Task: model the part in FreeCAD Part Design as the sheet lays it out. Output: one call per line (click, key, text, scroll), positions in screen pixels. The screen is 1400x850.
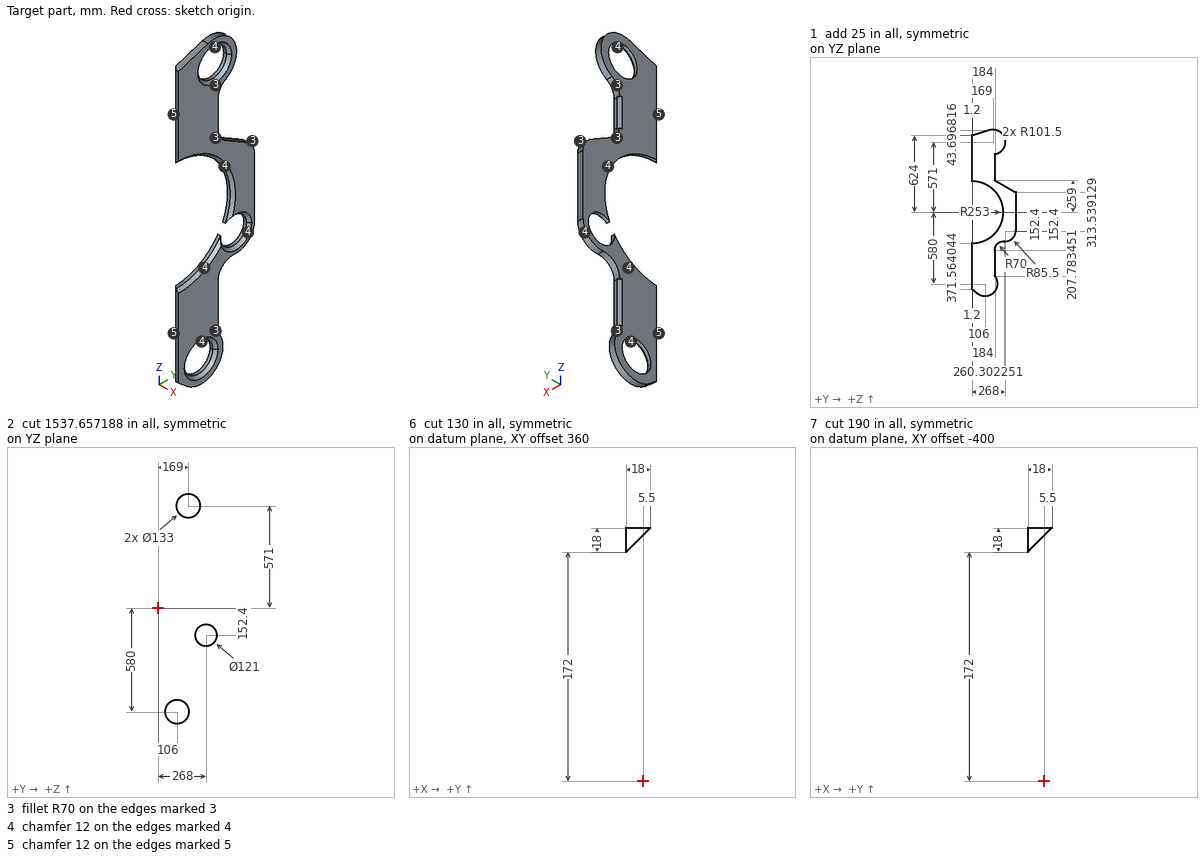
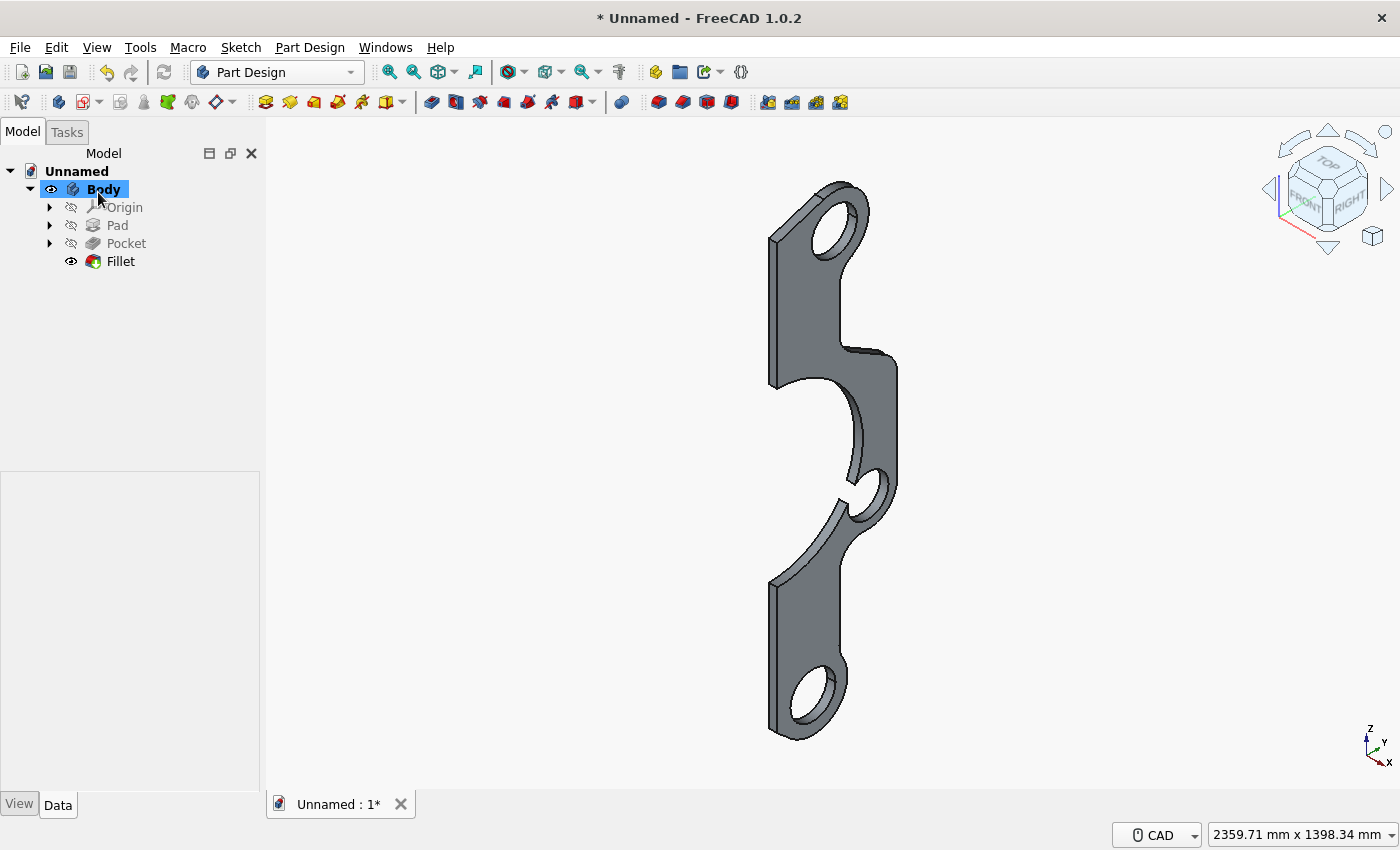
click(849, 392)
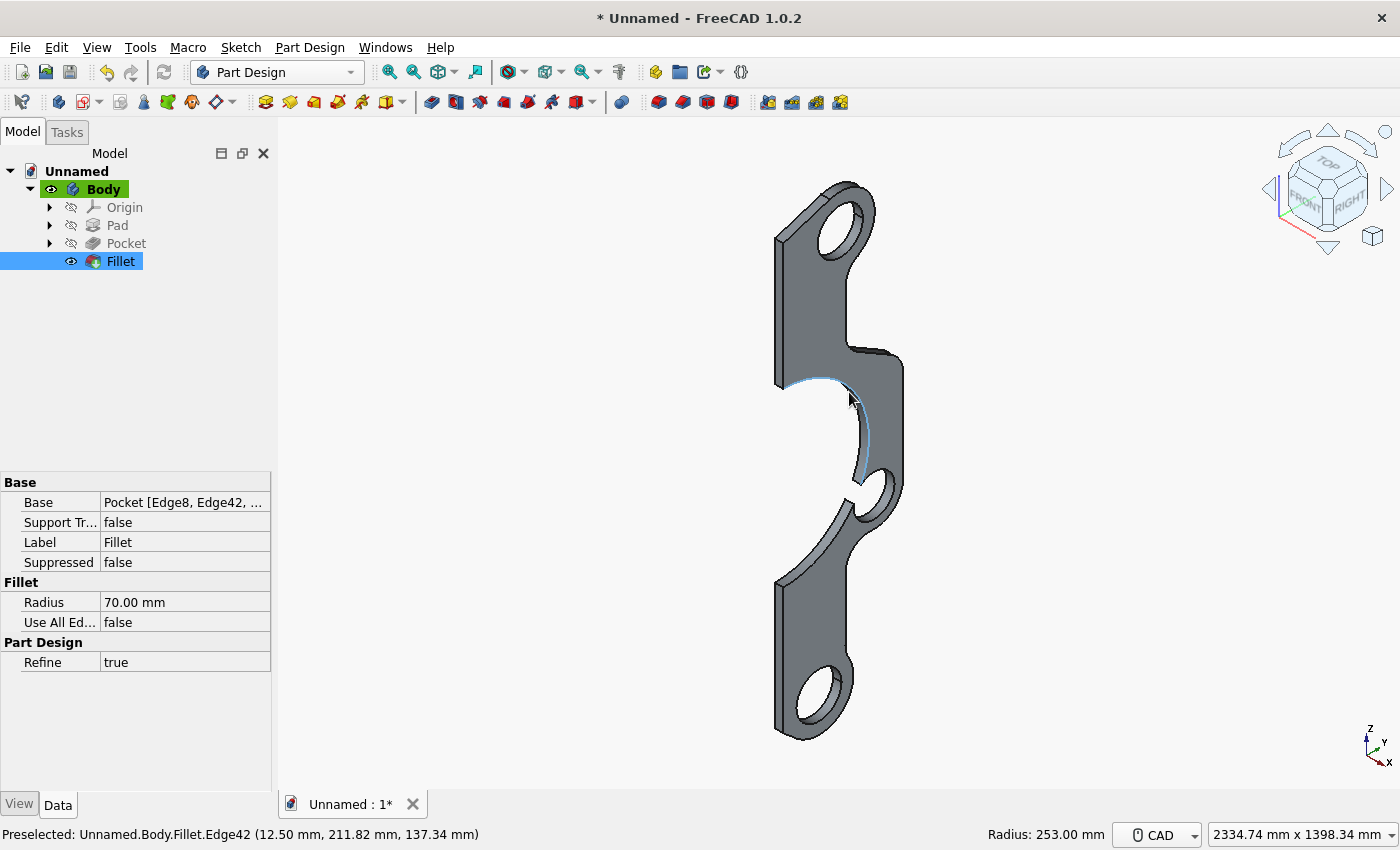
click(823, 552, ctrl)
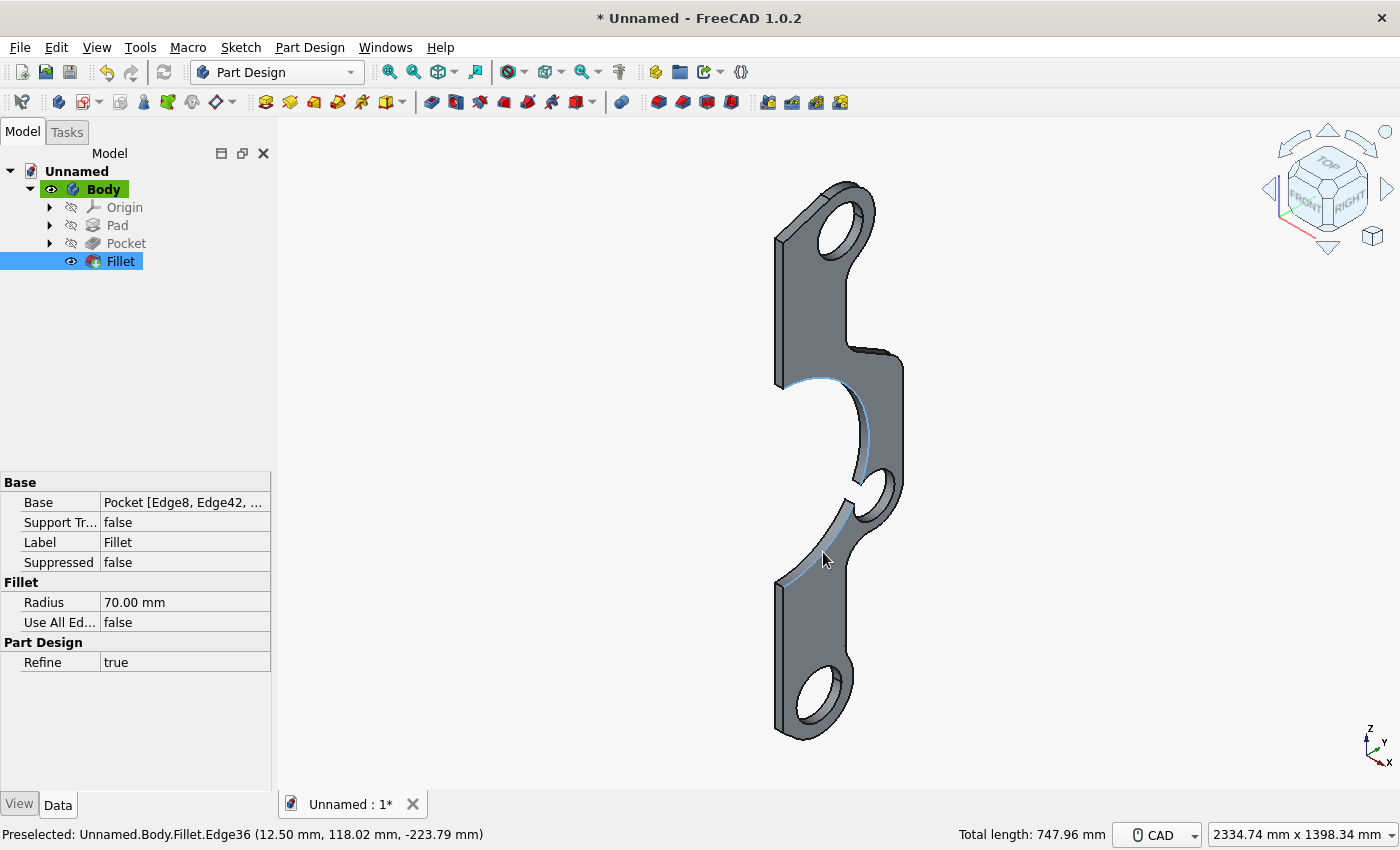
click(873, 519, ctrl)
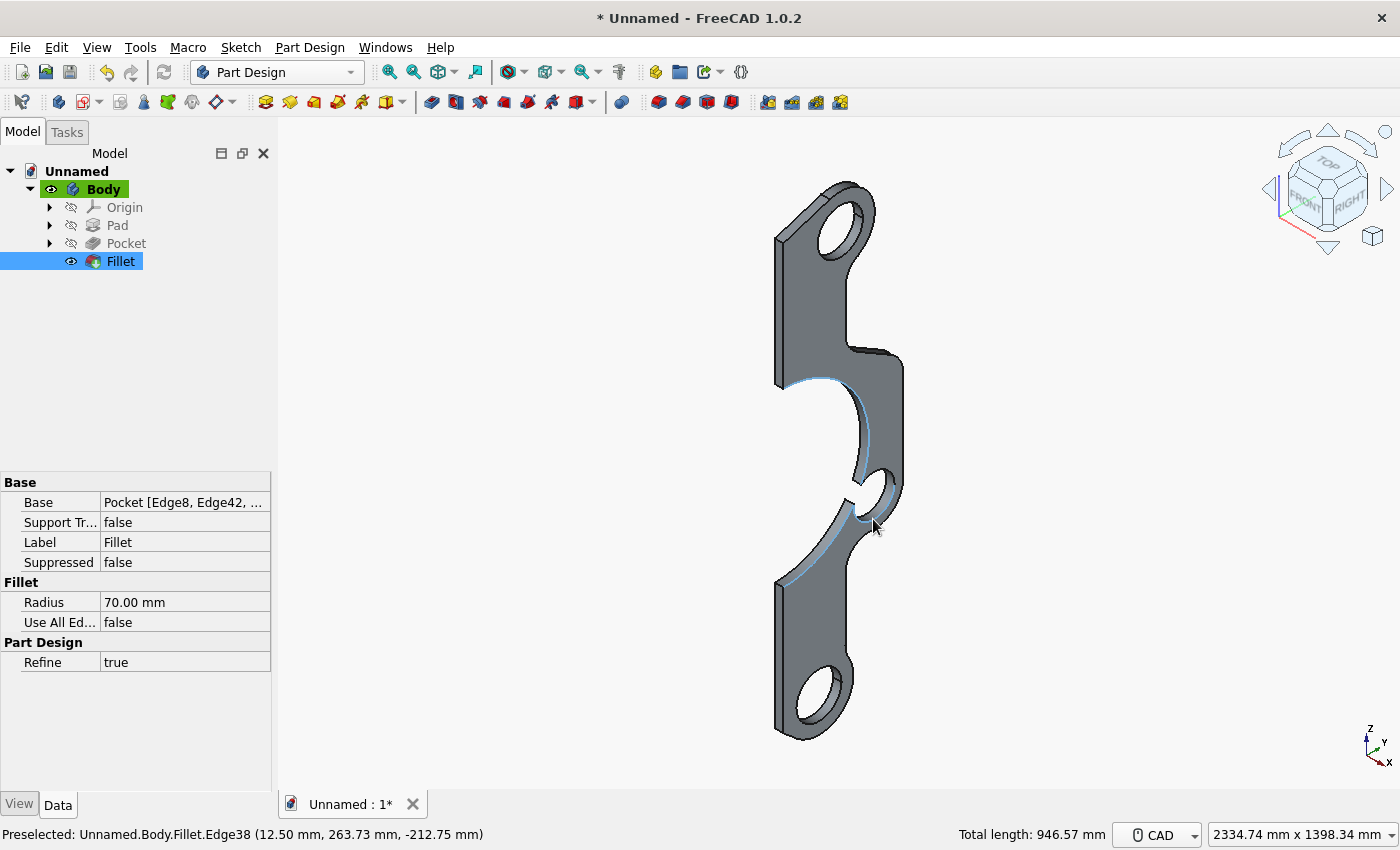
click(833, 259, ctrl)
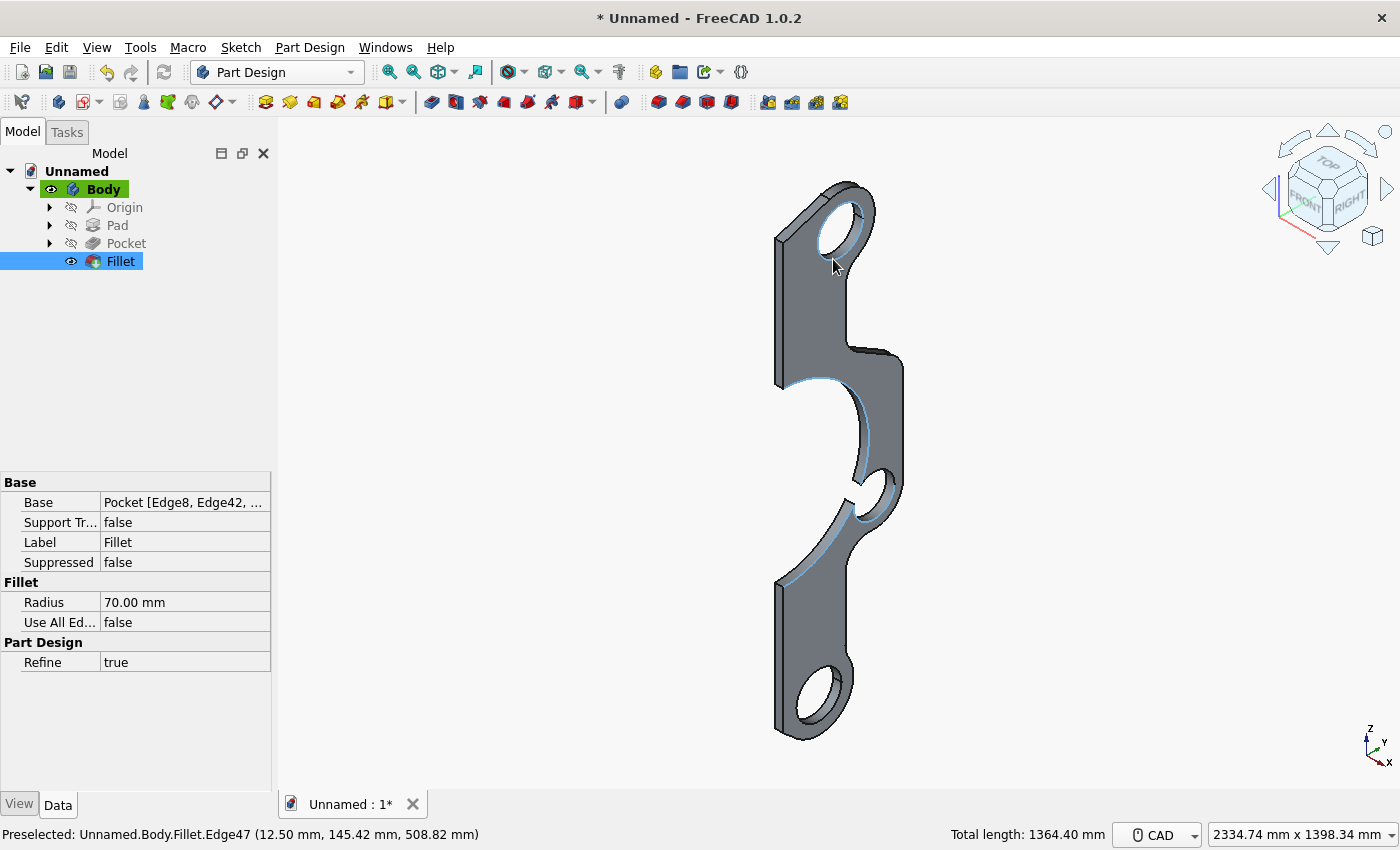
click(801, 720, ctrl)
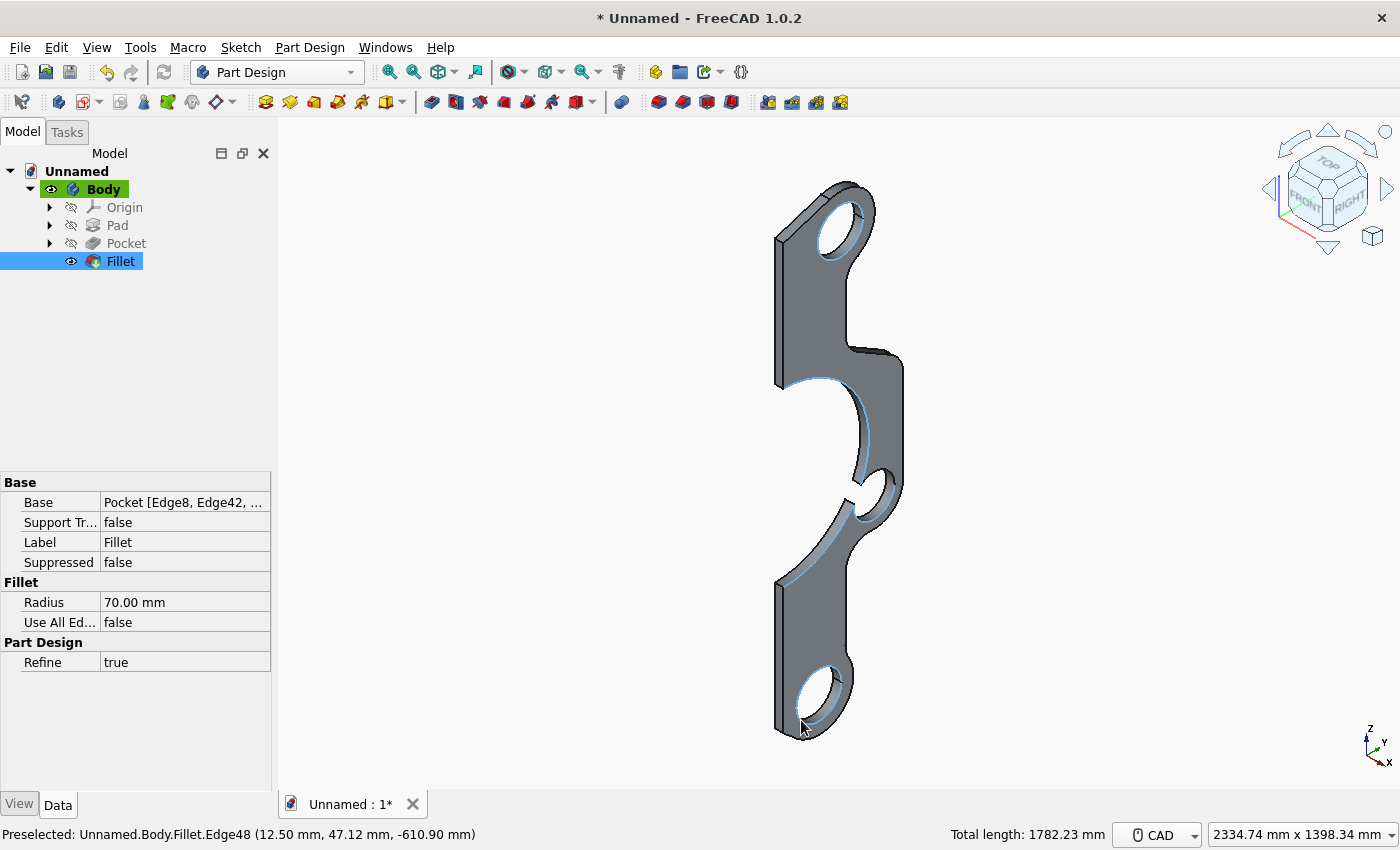
click(684, 102)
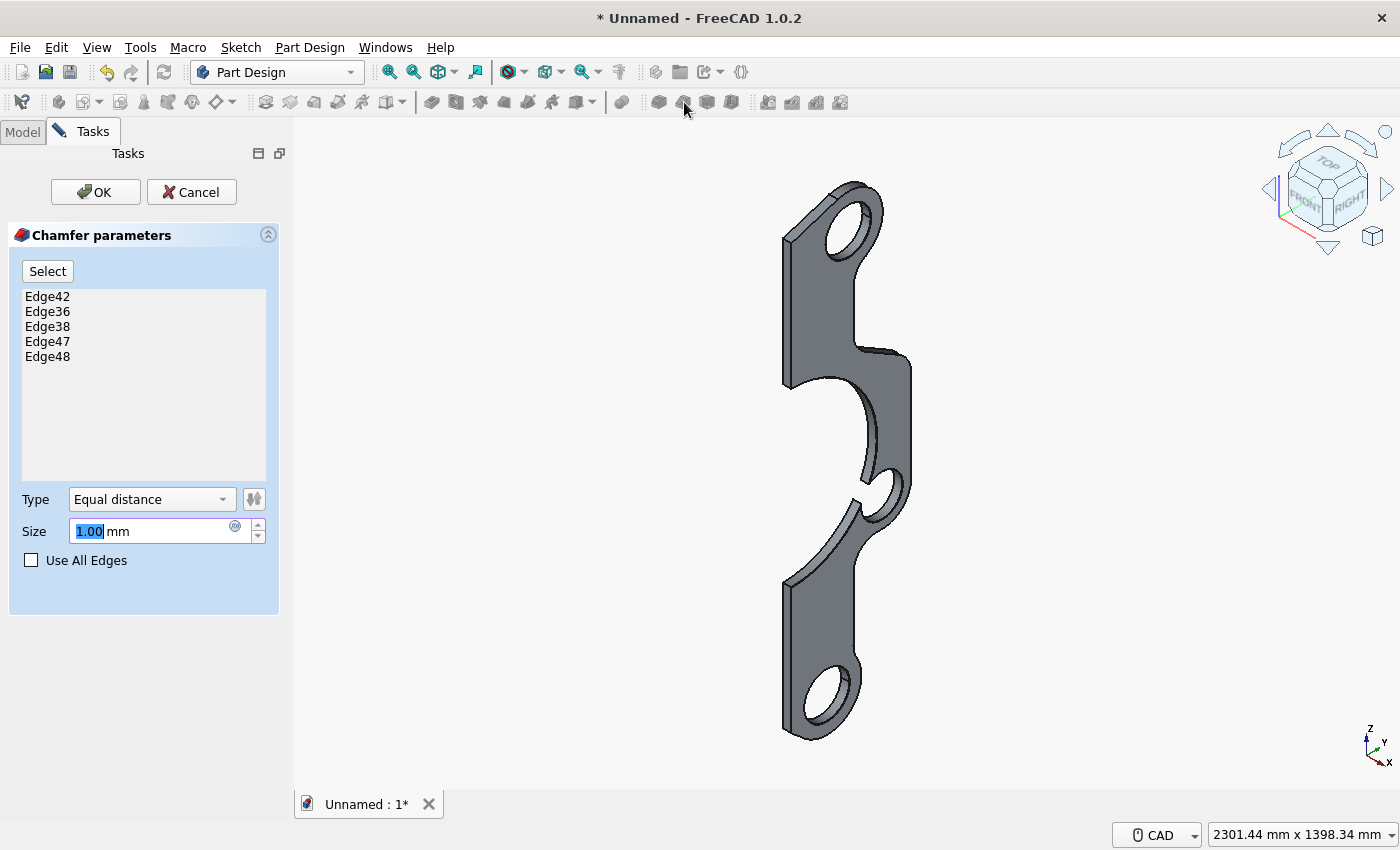
text(12)
key(Tab)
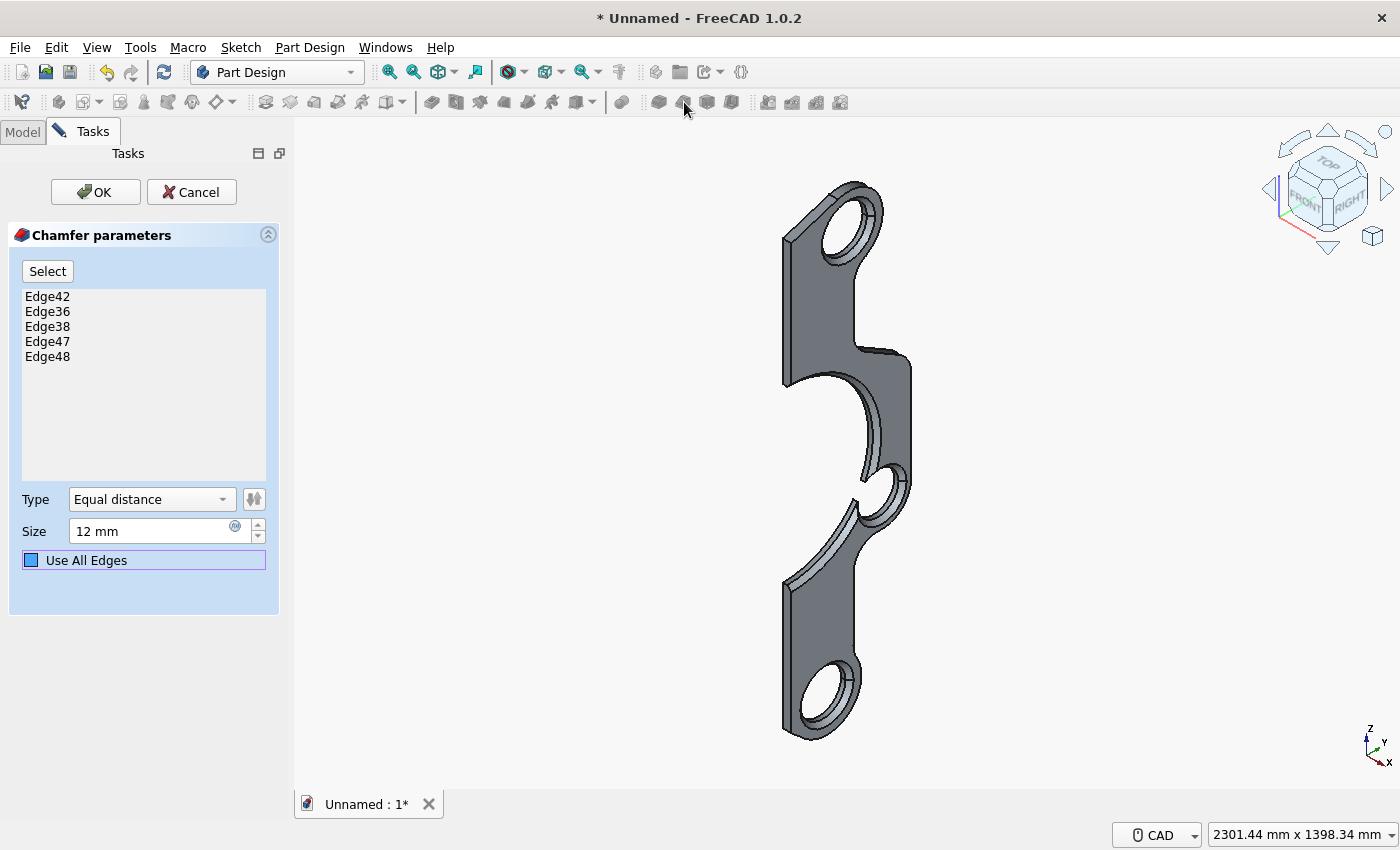
click(96, 192)